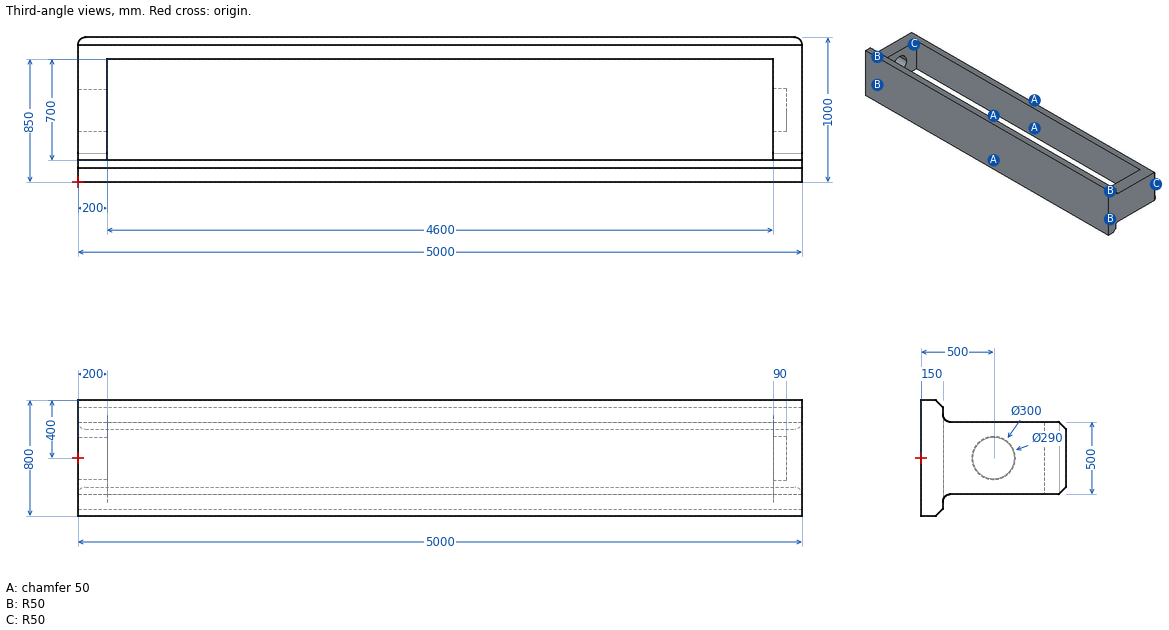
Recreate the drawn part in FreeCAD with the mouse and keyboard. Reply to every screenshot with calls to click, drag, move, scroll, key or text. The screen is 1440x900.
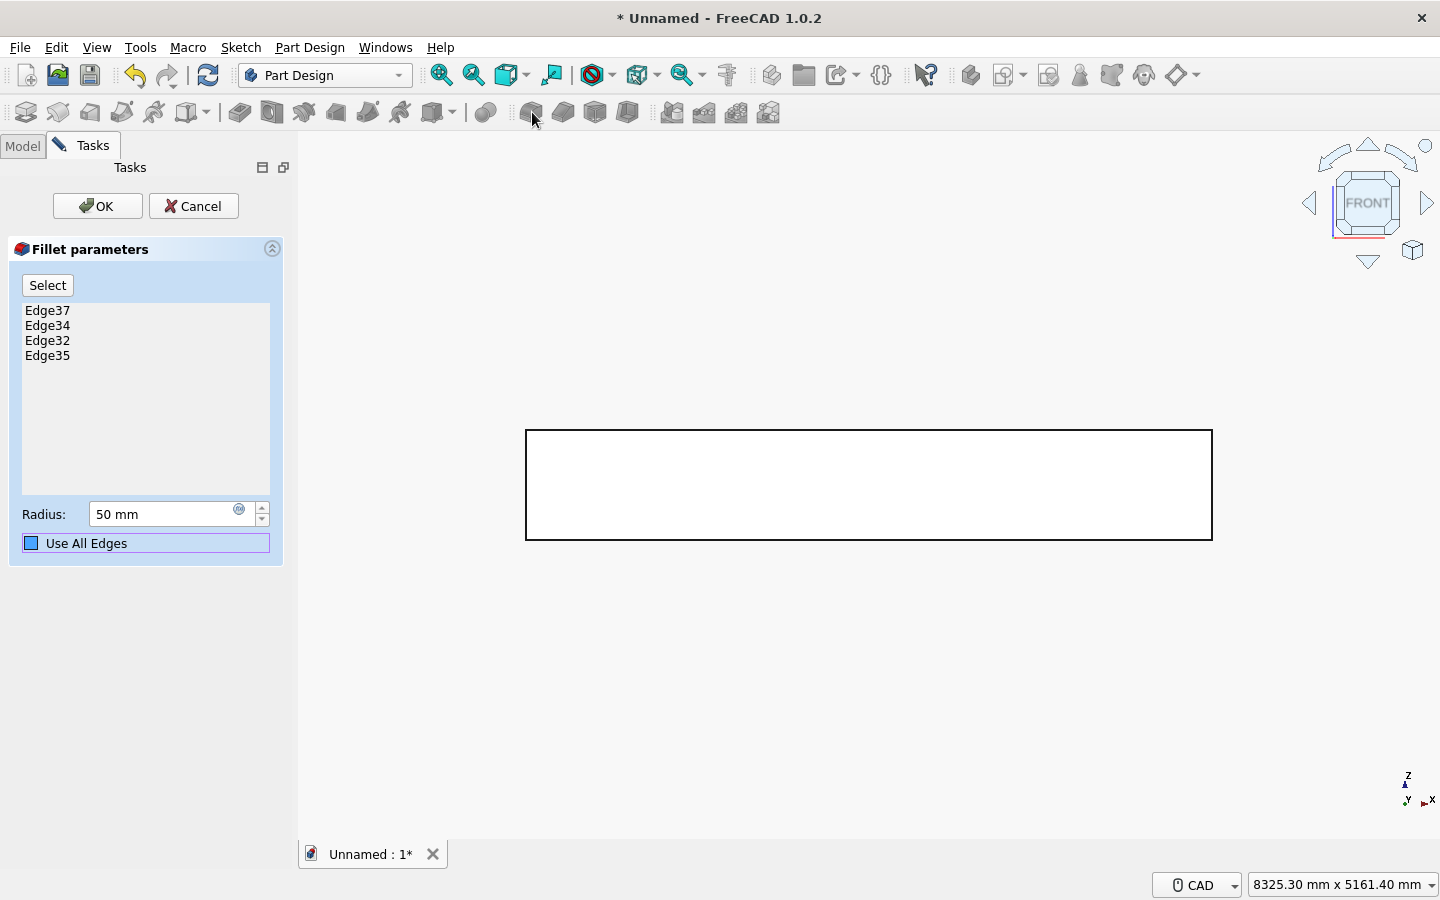
click(98, 206)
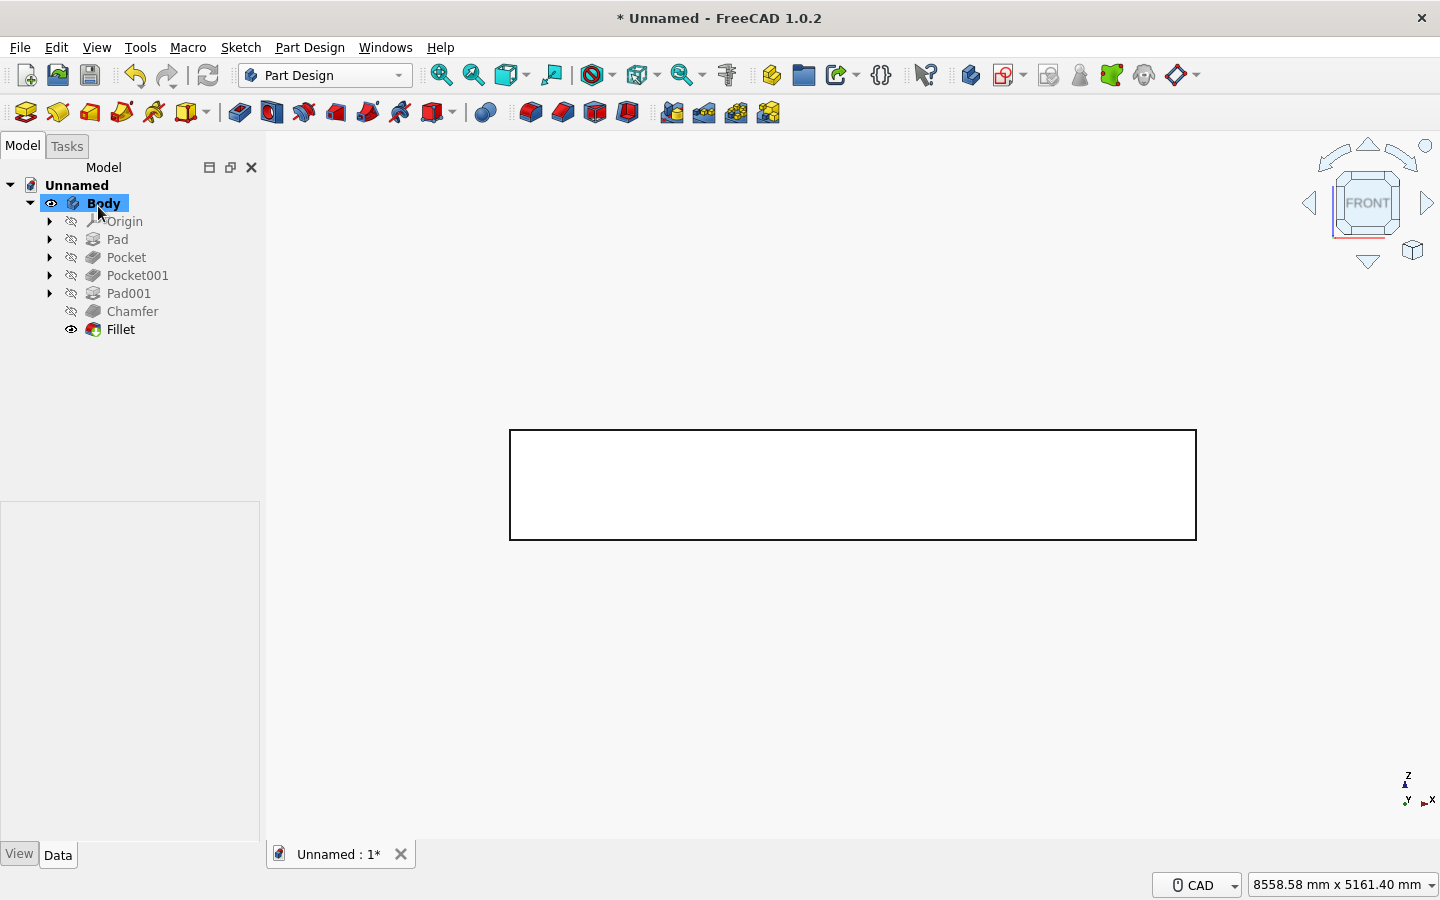
key(0)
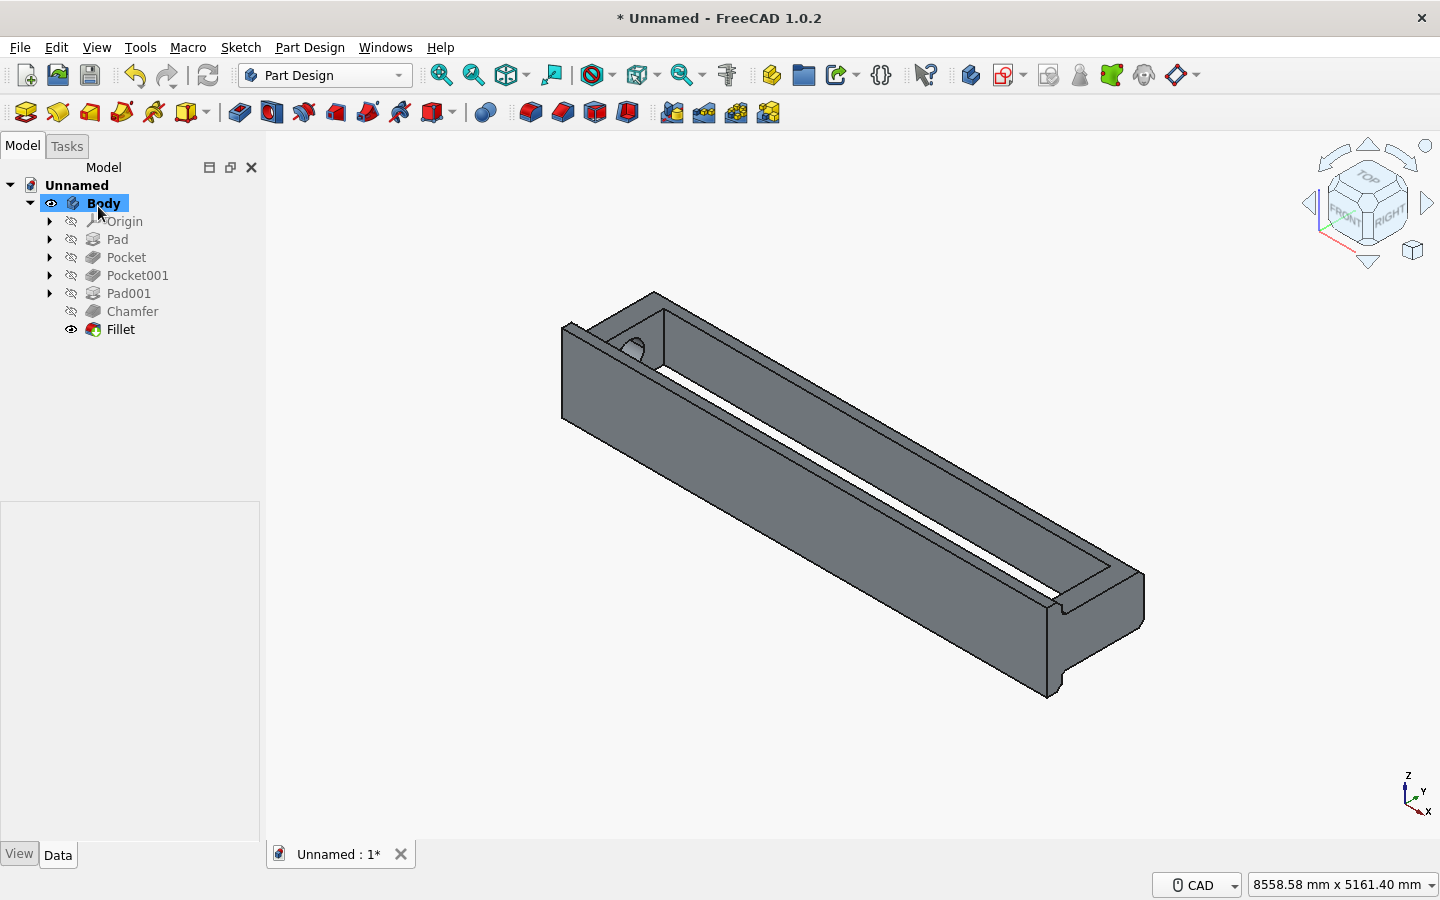
key(2)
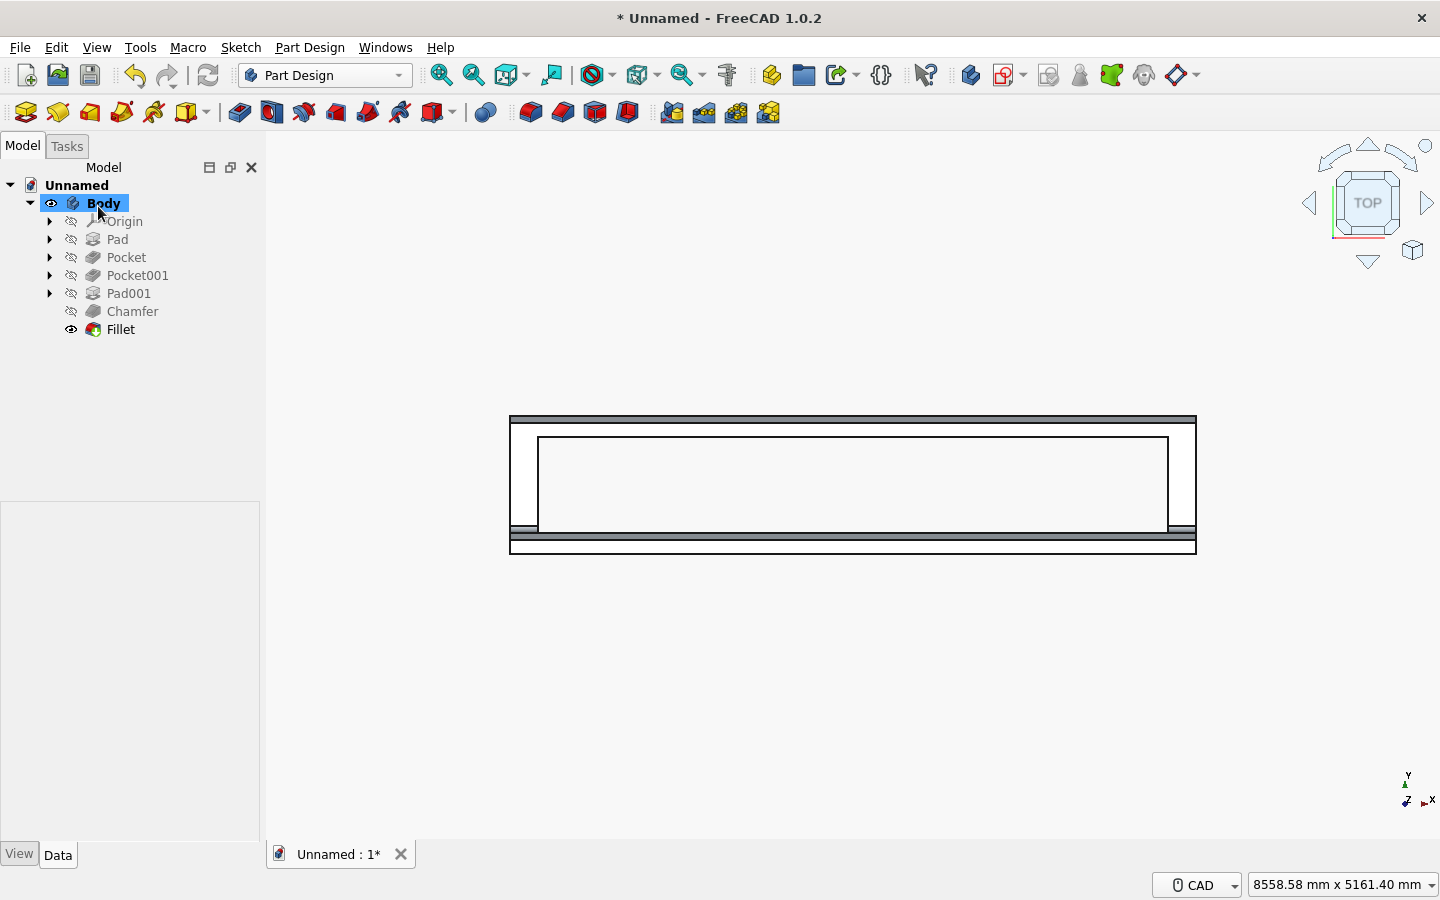
key(1)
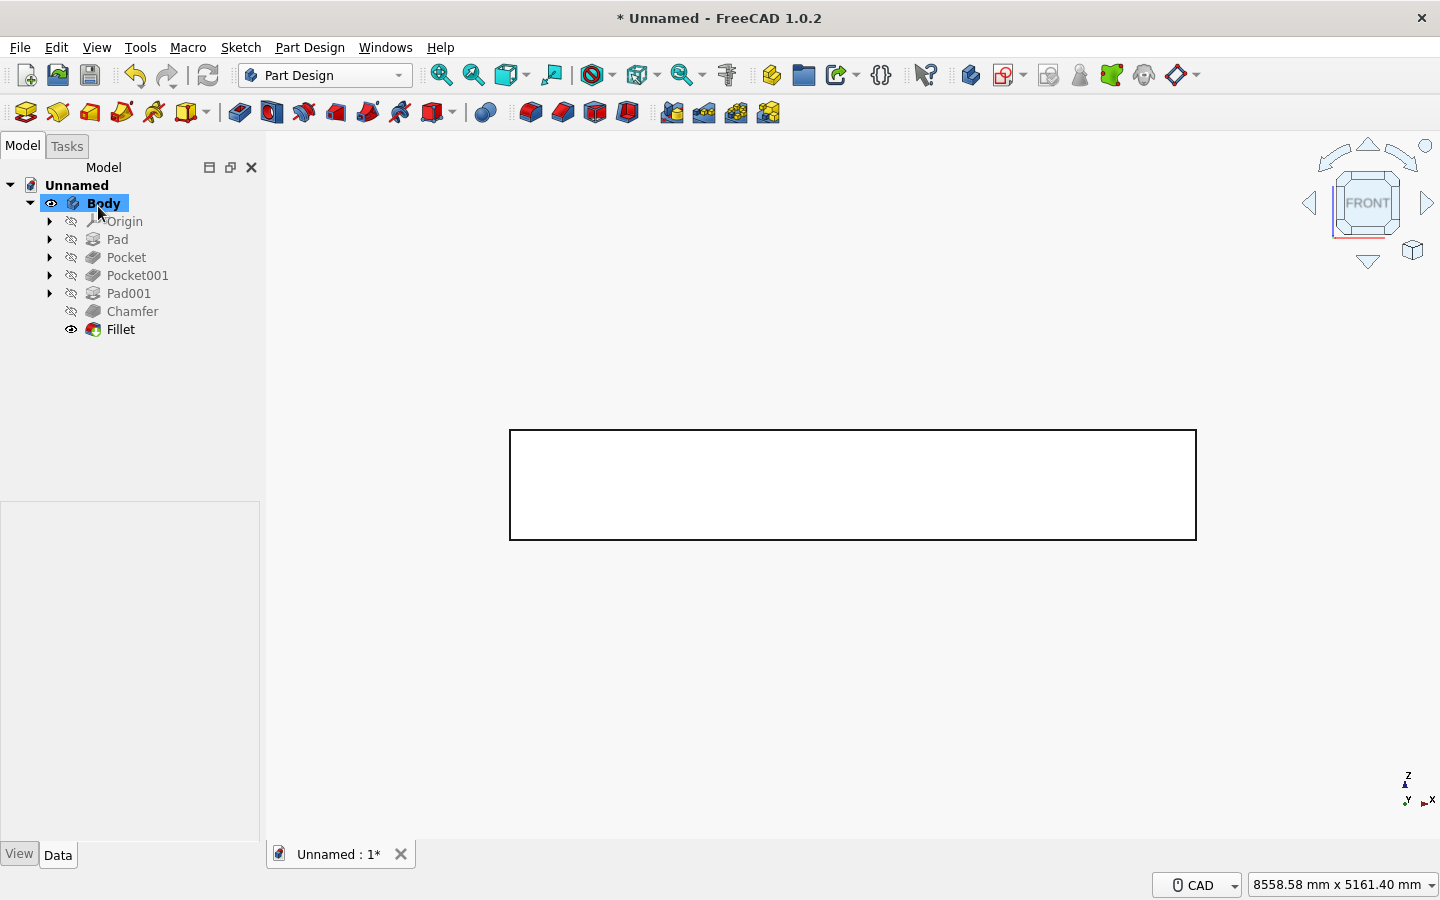
key(3)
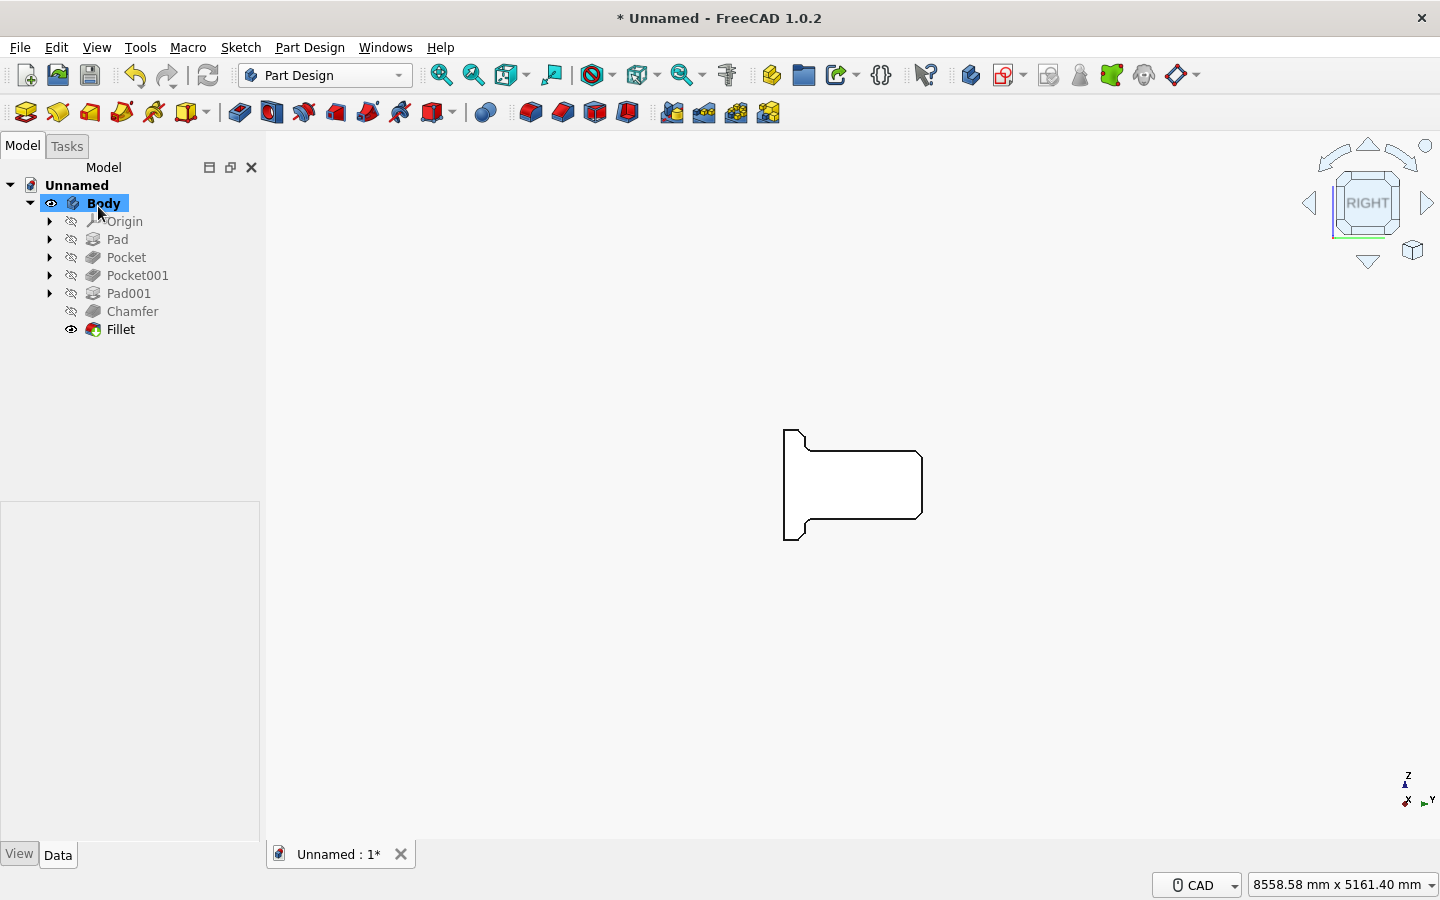
key(v)
key(f)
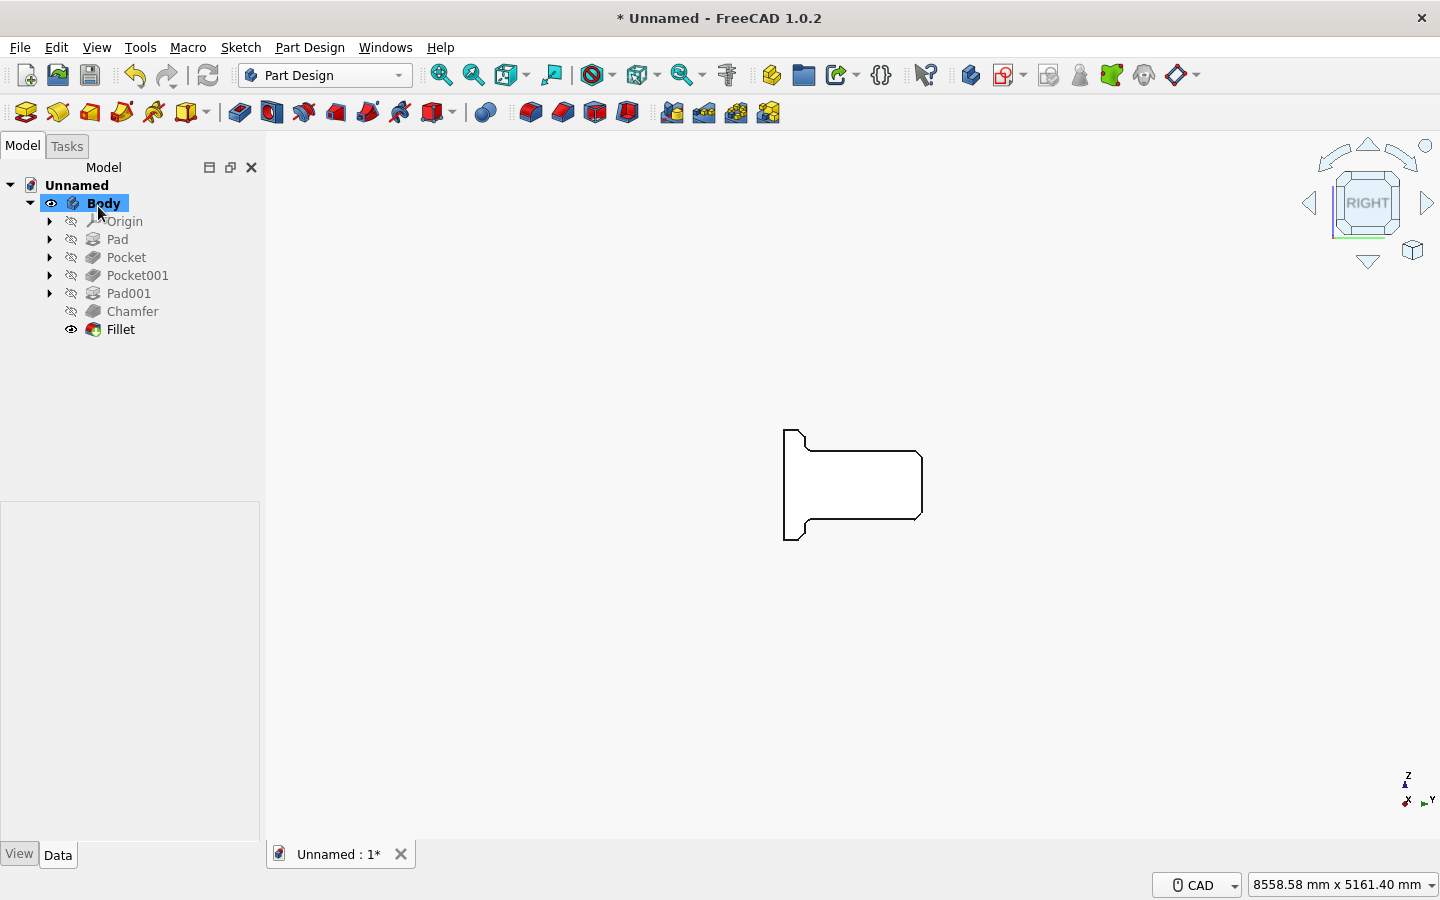
click(922, 484)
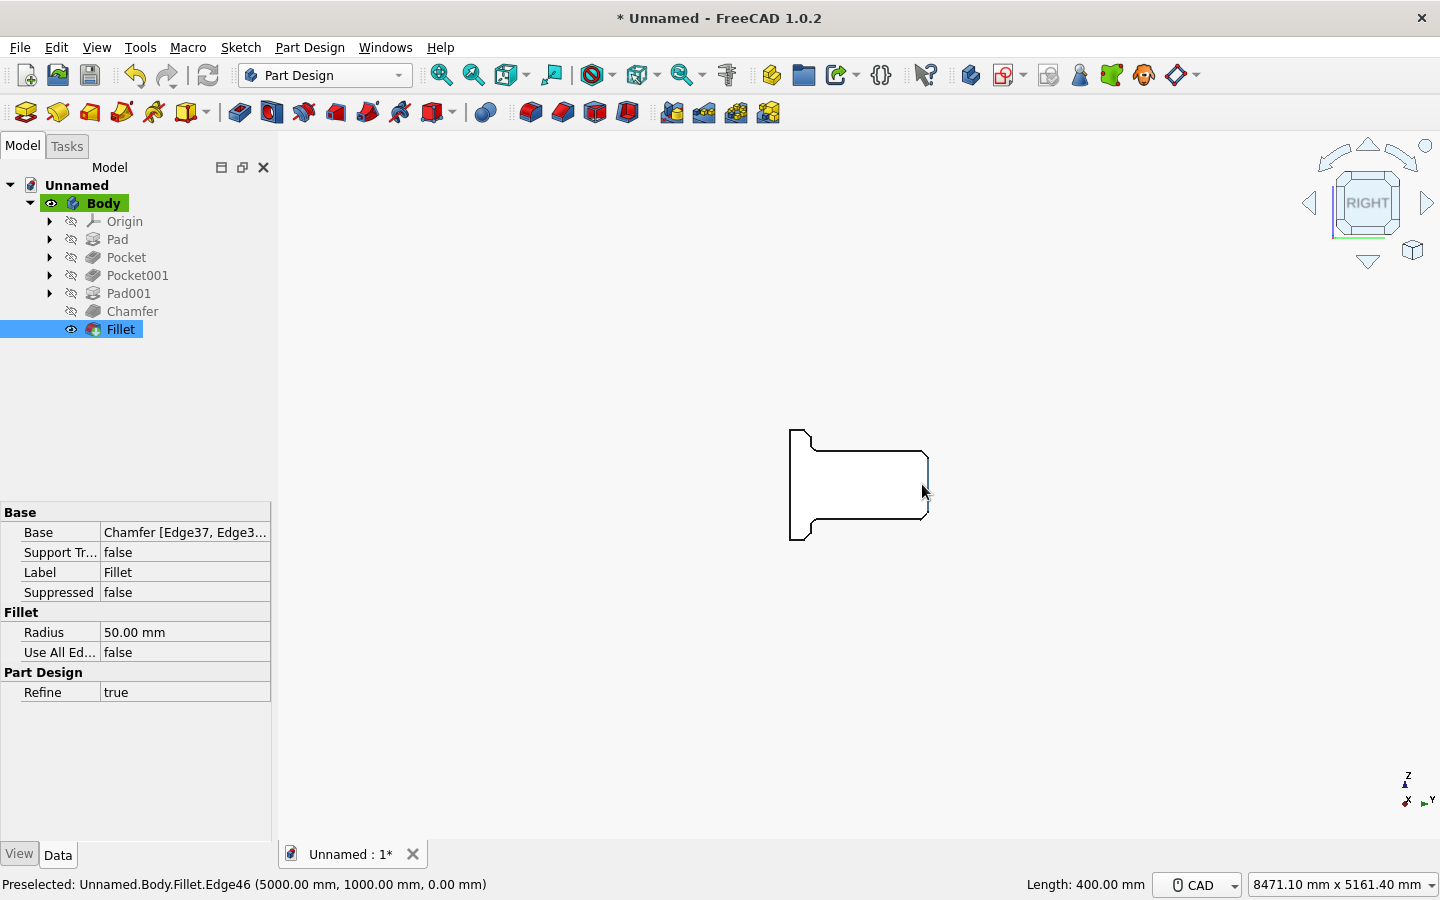
key(5)